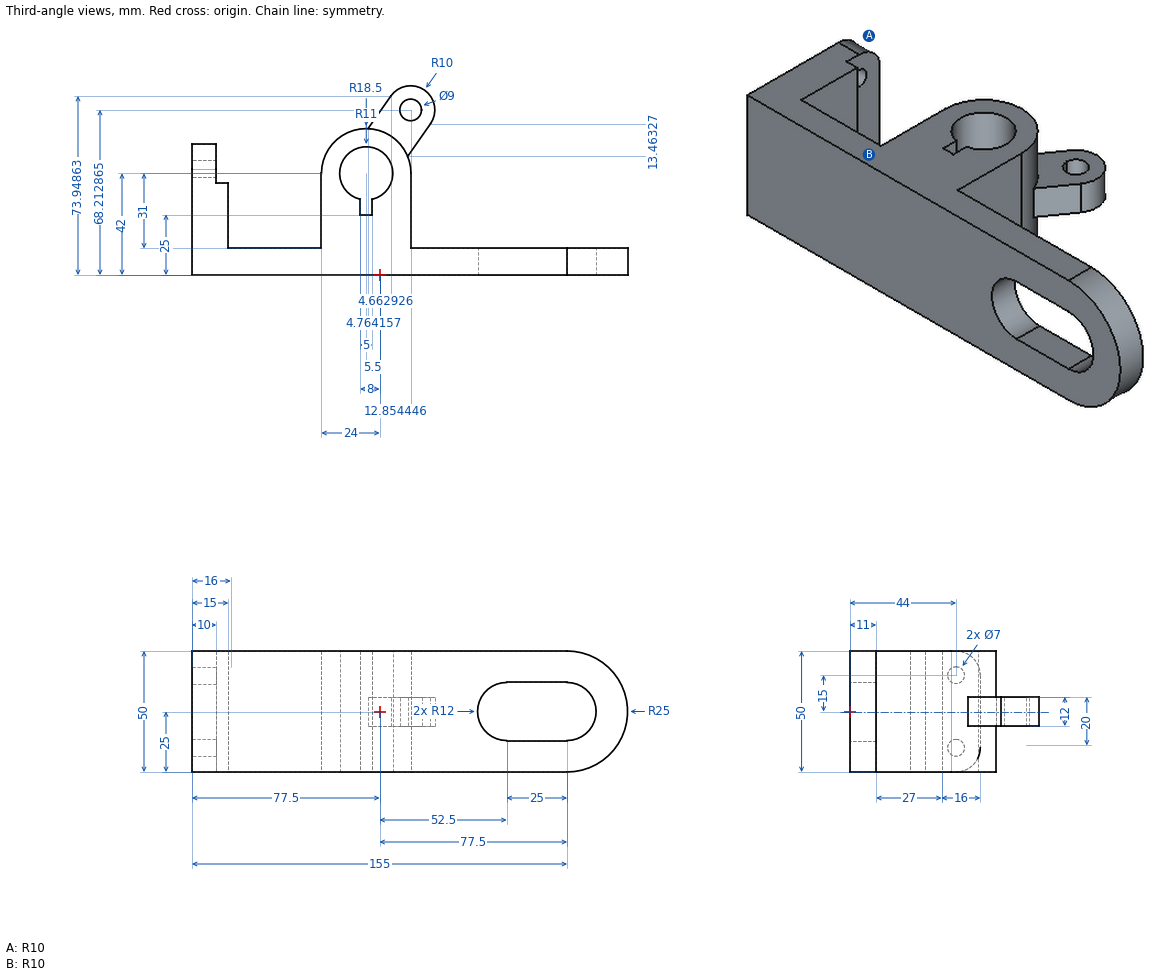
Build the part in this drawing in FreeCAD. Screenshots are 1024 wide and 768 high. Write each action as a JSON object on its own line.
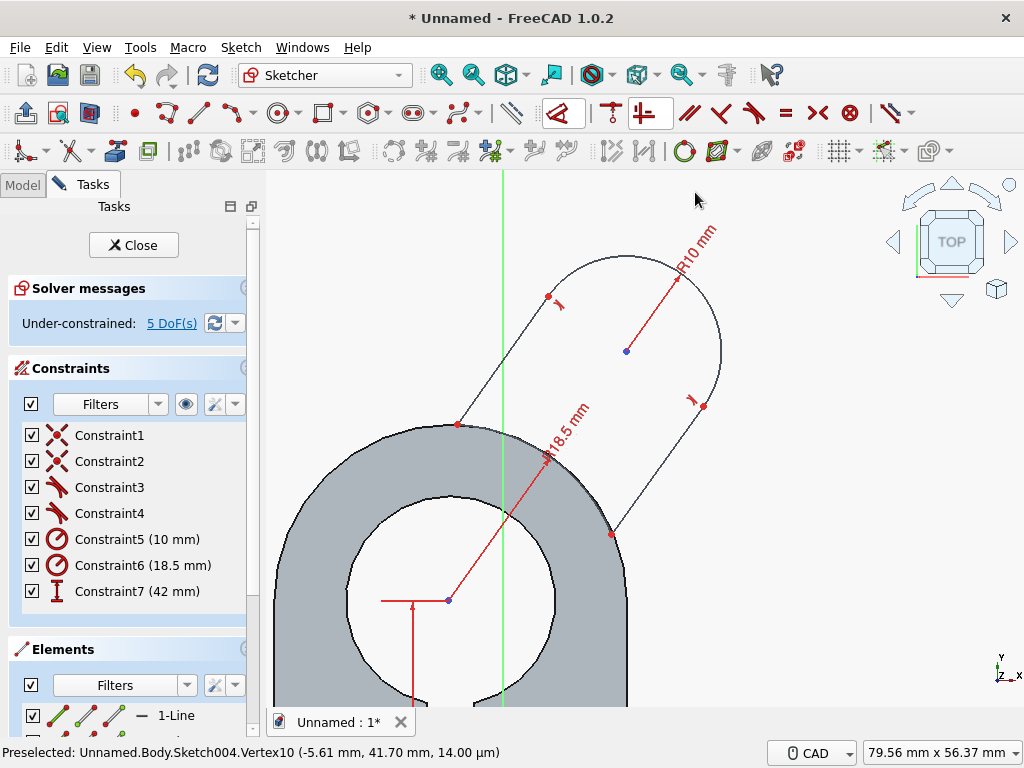
{"action": "left_click", "coordinate": [448, 601]}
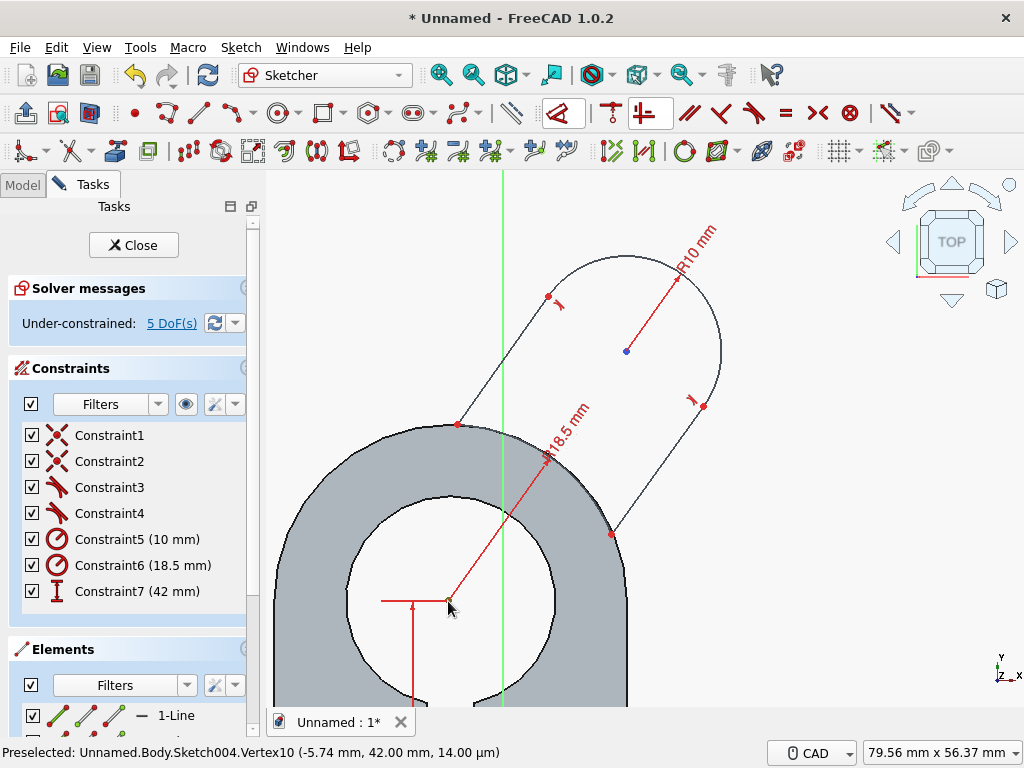
{"action": "key", "text": "l"}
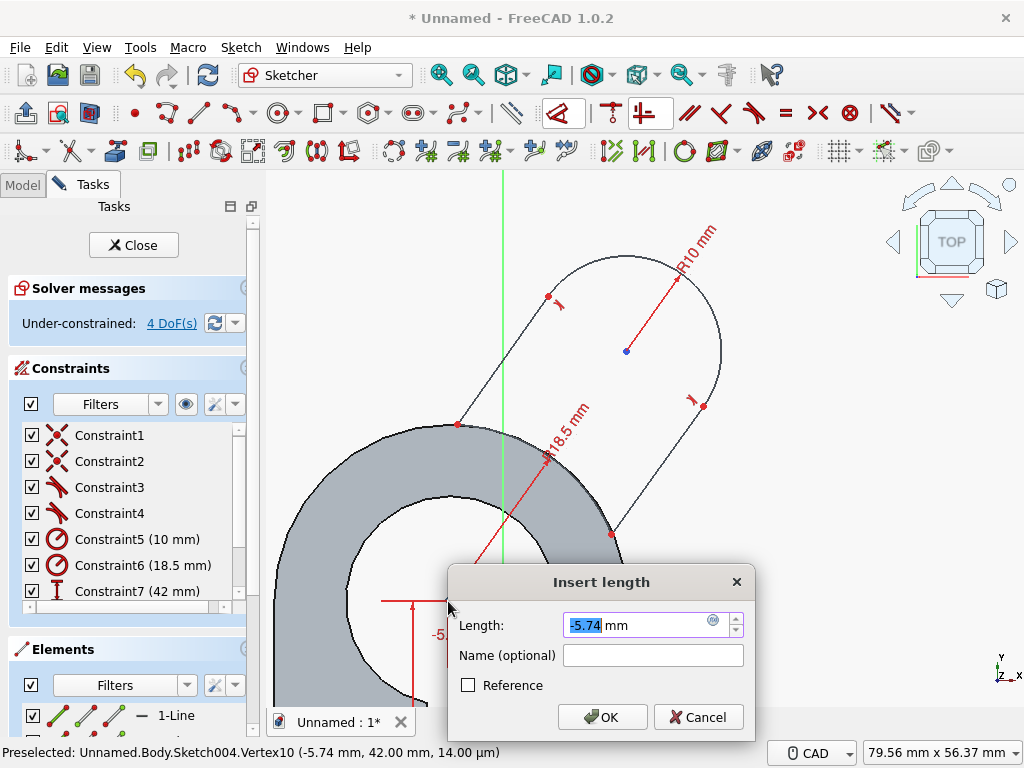
{"action": "type", "text": "-5.5"}
{"action": "key", "text": "Return"}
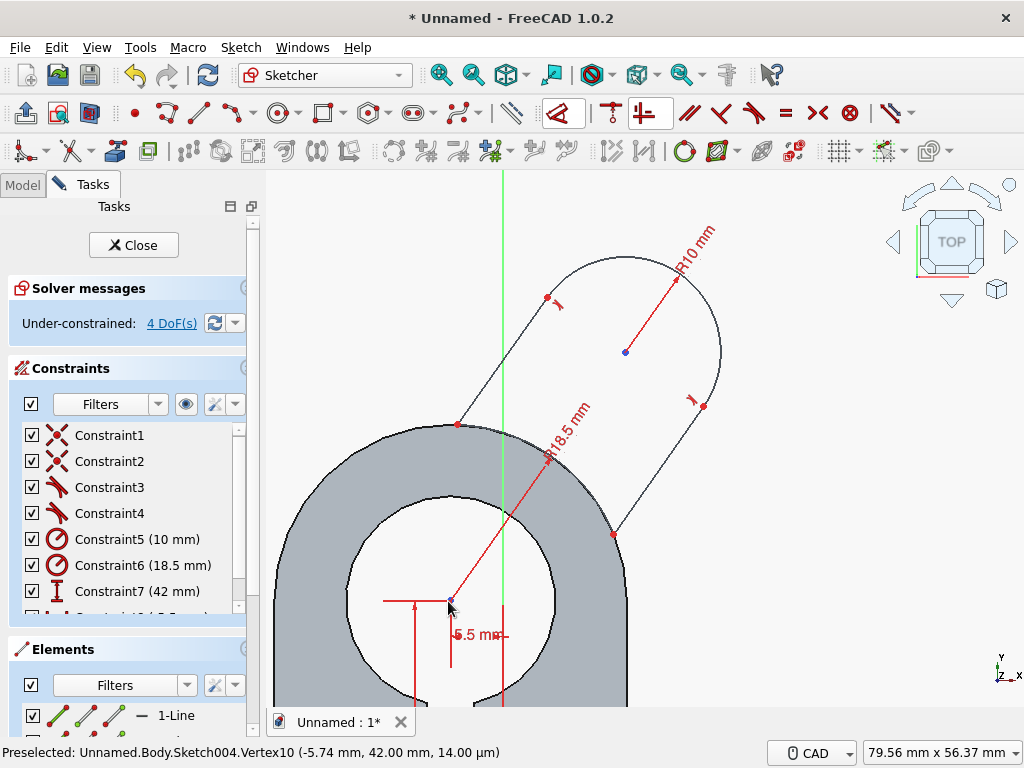
{"action": "left_click", "coordinate": [548, 297]}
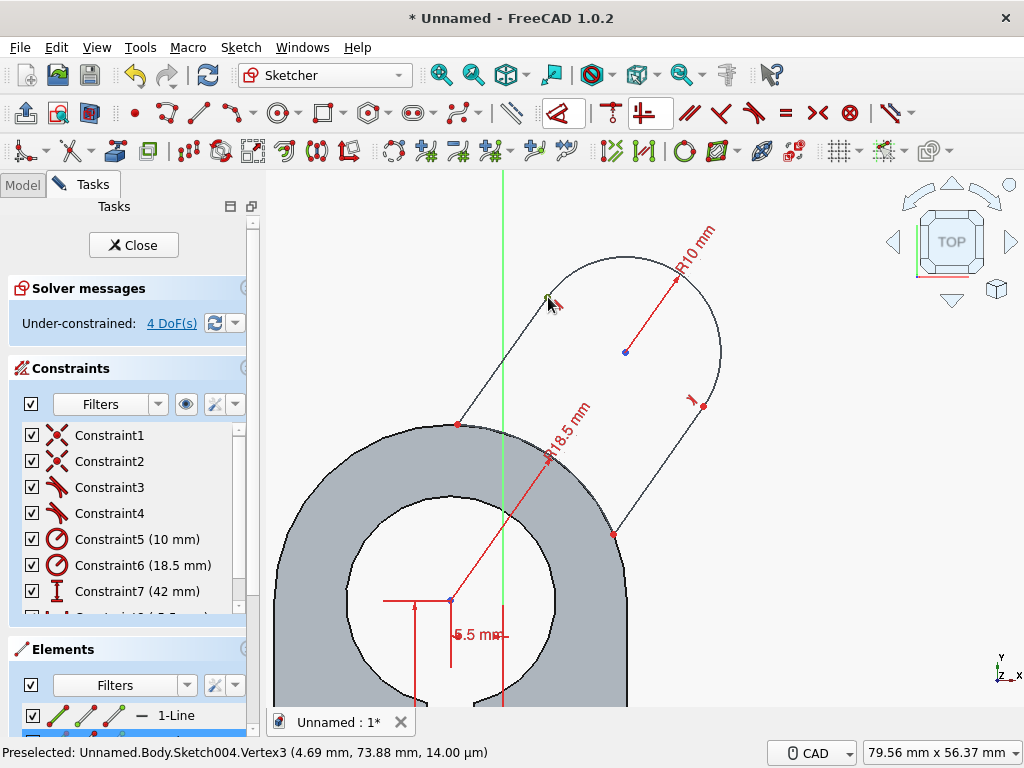
{"action": "key", "text": "l"}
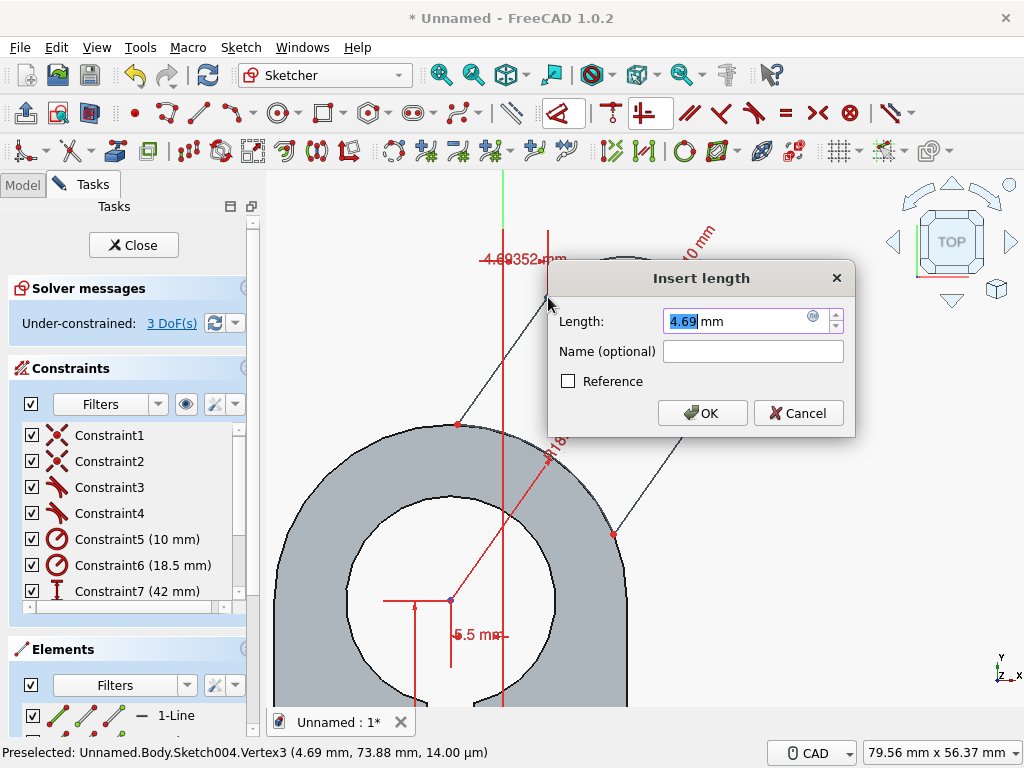
{"action": "type", "text": "4.662926"}
{"action": "key", "text": "Return"}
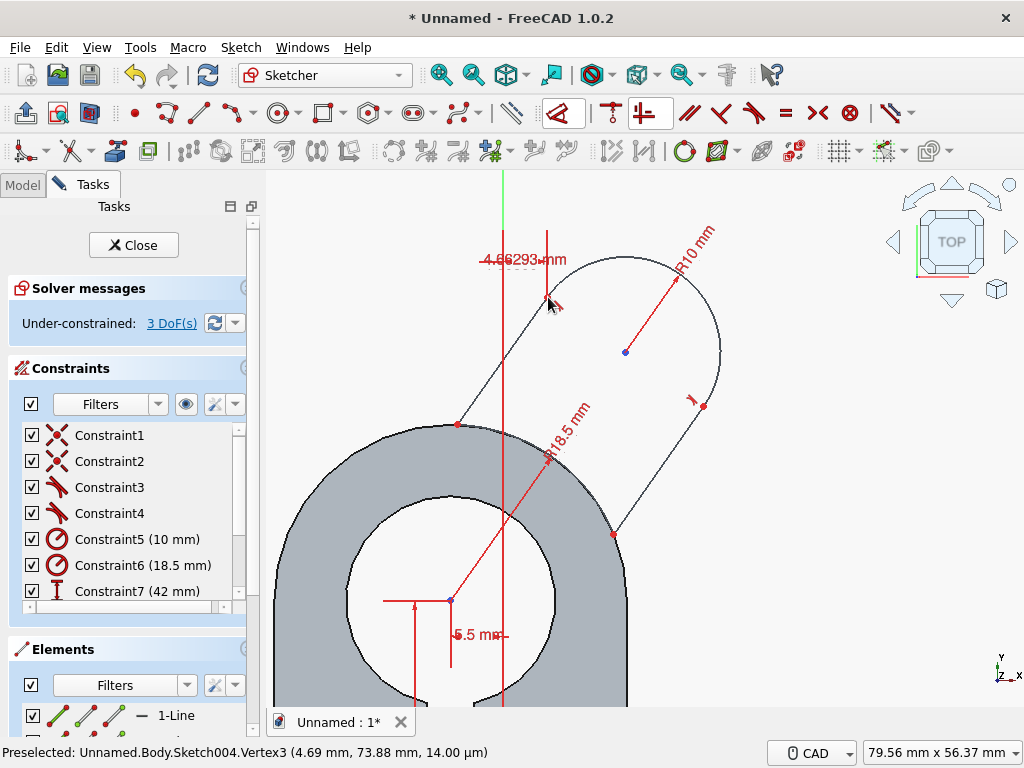
{"action": "left_click", "coordinate": [547, 297]}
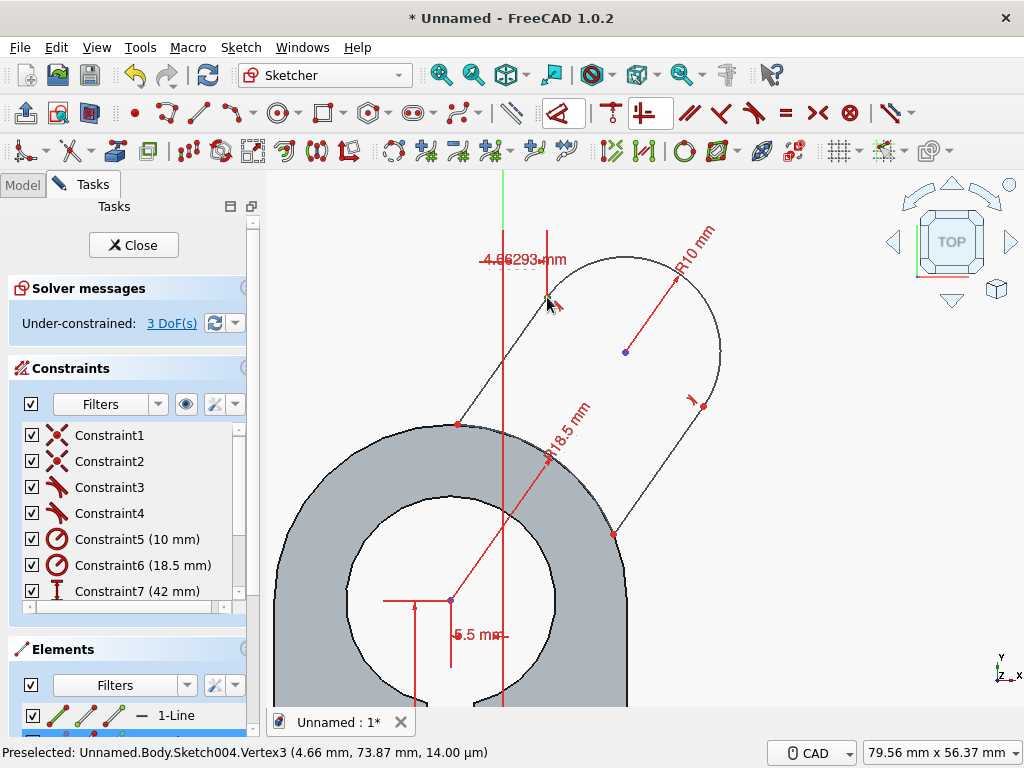
{"action": "key", "text": "i"}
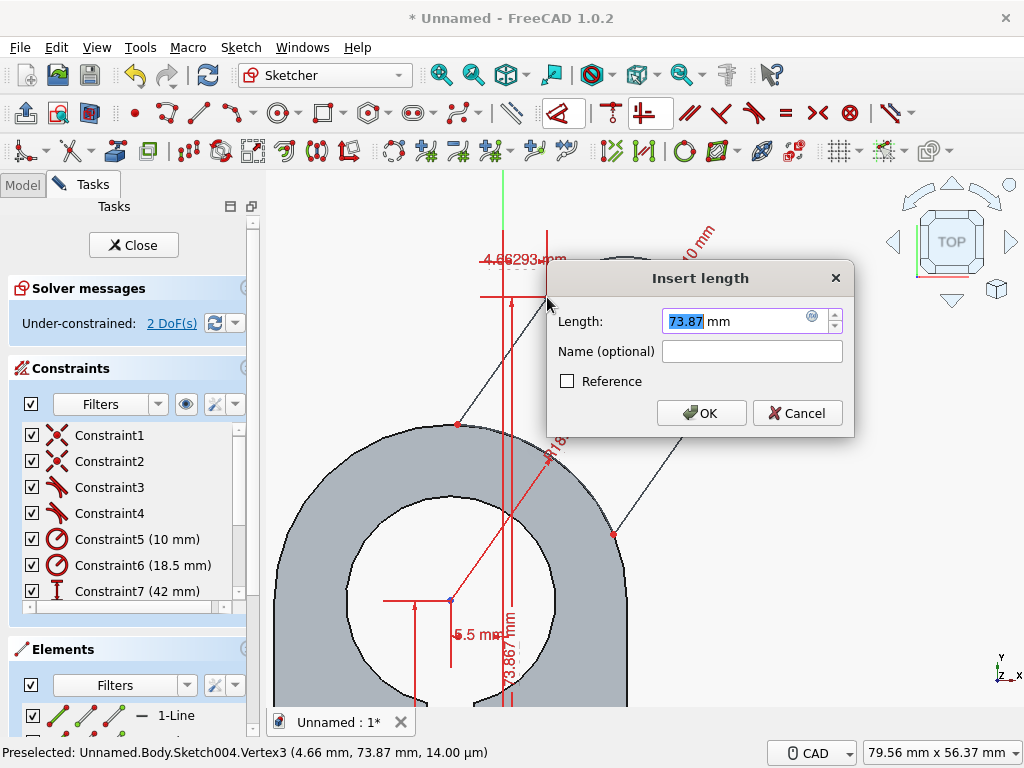
{"action": "type", "text": "73.94863"}
{"action": "key", "text": "Return"}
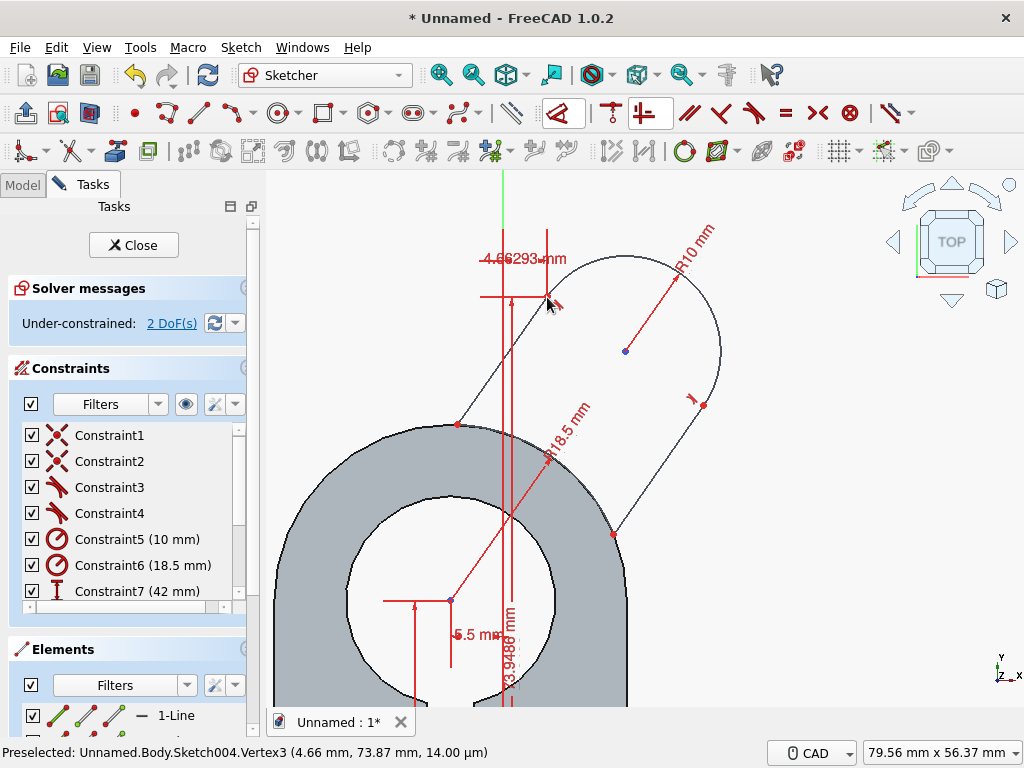
{"action": "left_click", "coordinate": [457, 425]}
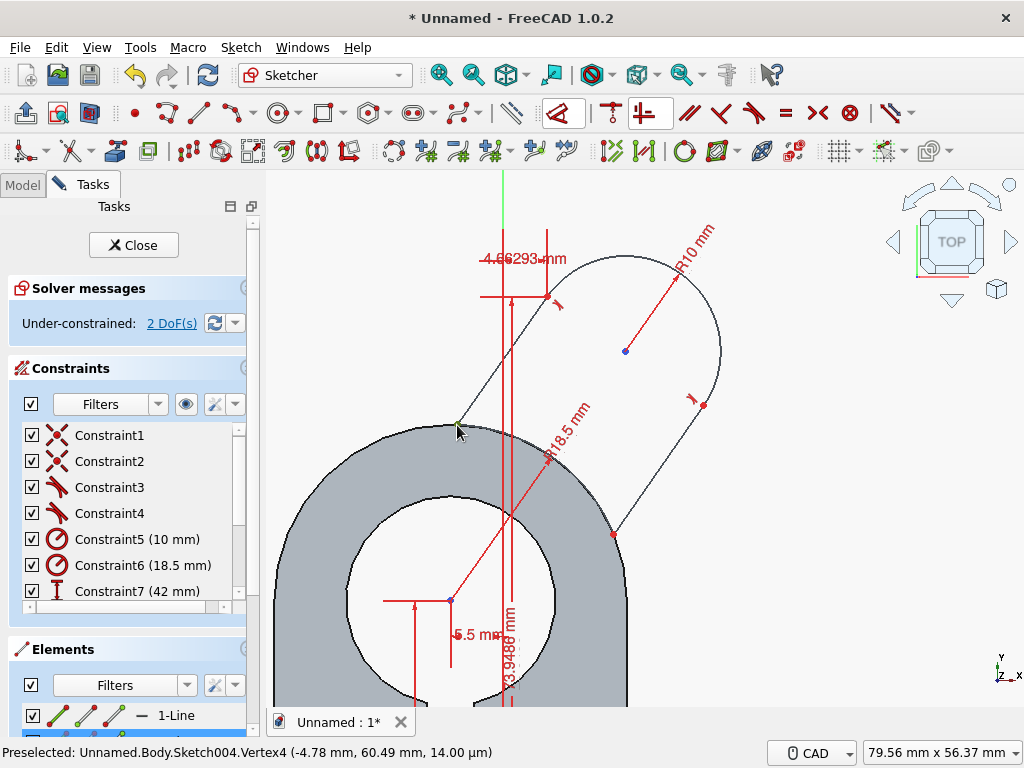
{"action": "left_click", "coordinate": [580, 114]}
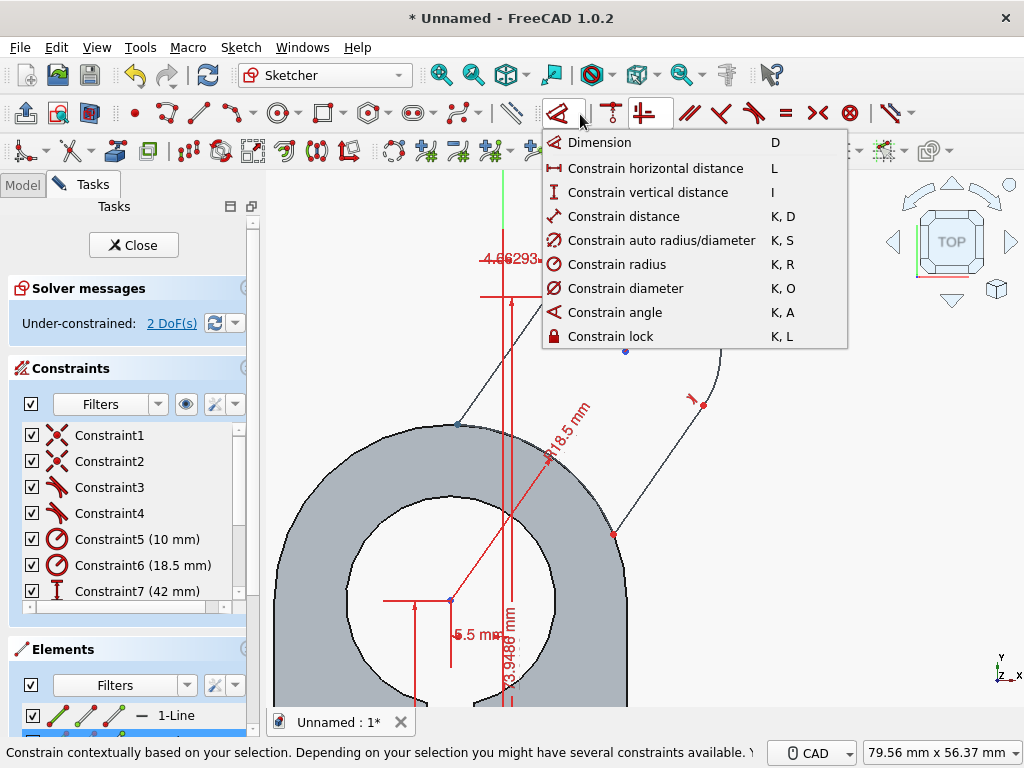
{"action": "left_click", "coordinate": [695, 168]}